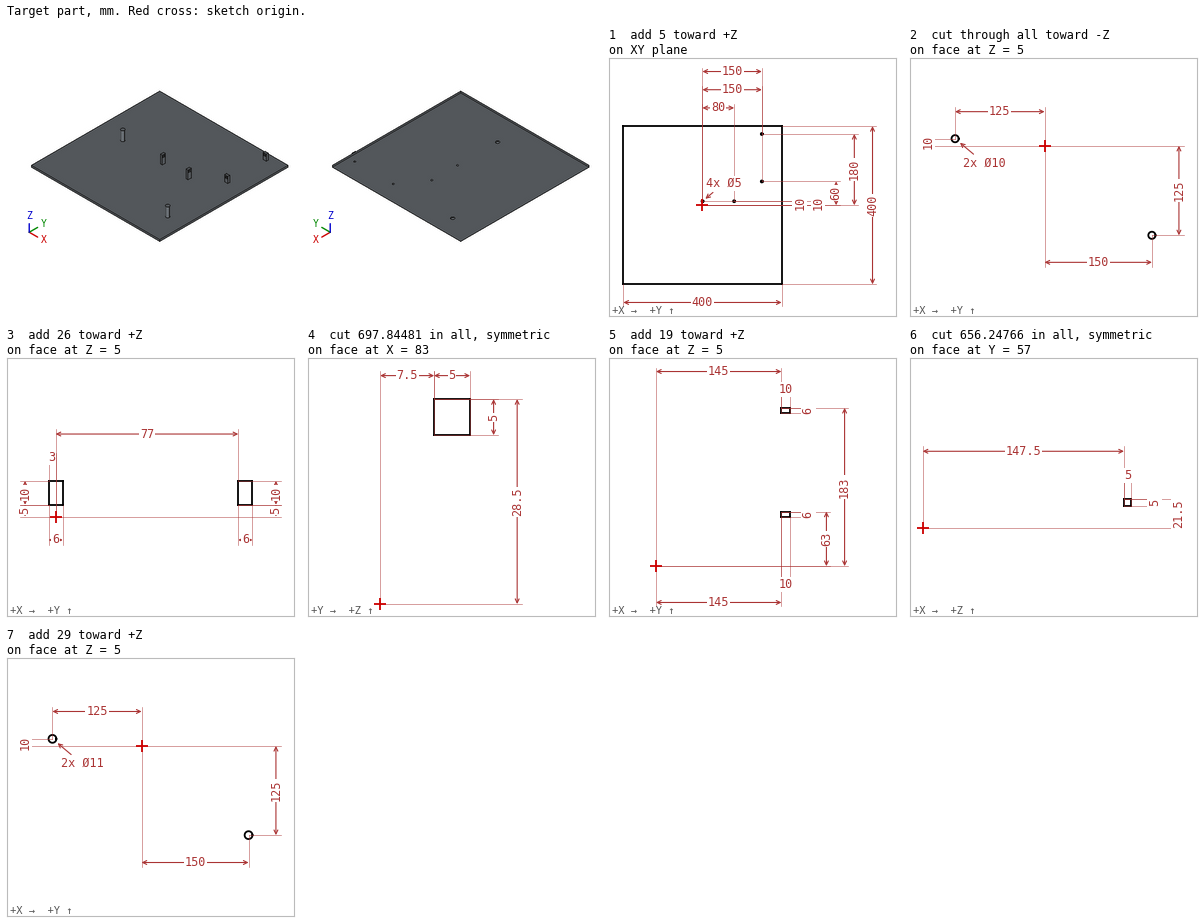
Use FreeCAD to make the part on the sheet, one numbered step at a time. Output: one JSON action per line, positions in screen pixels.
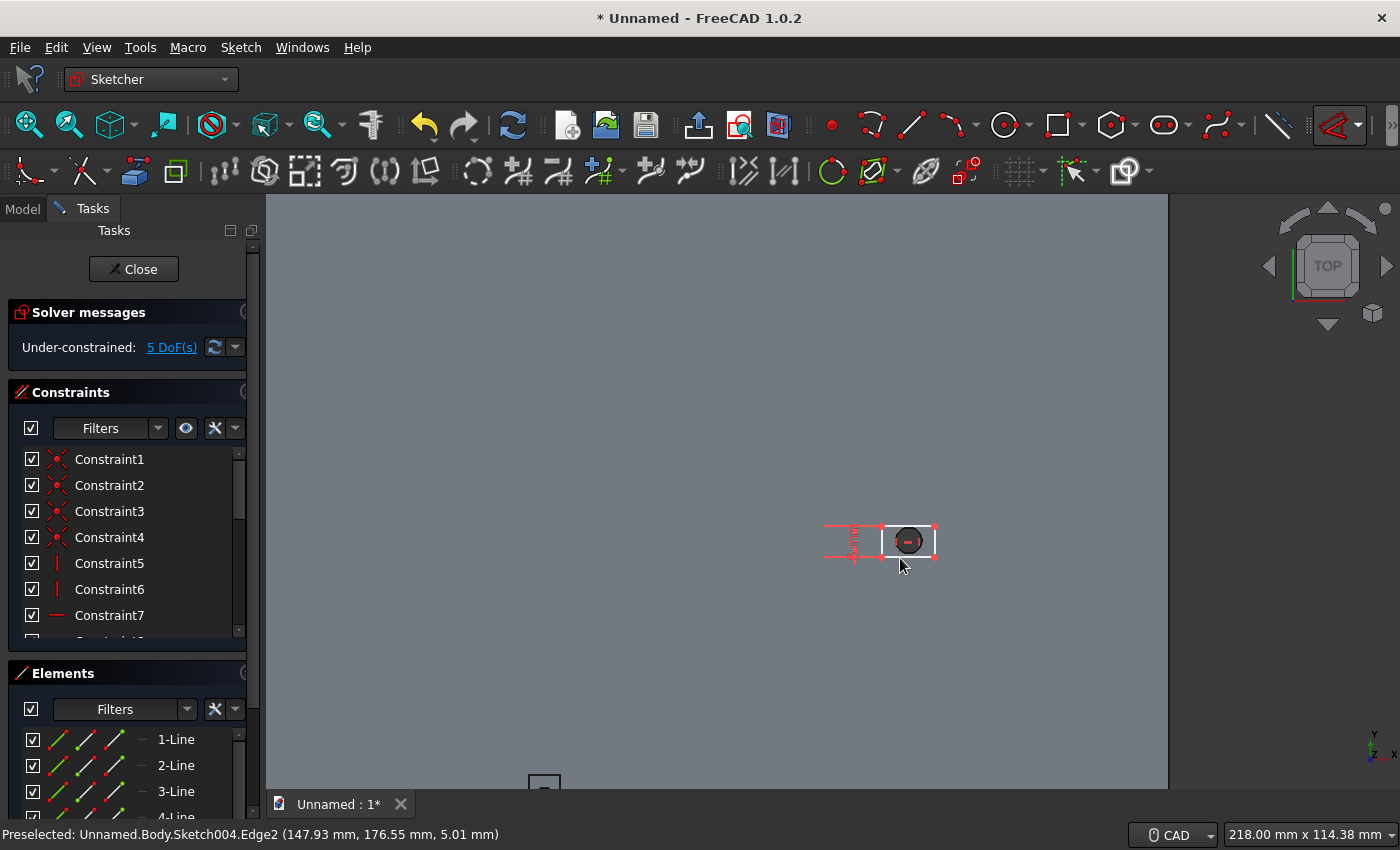
{"action": "left_click", "coordinate": [898, 557]}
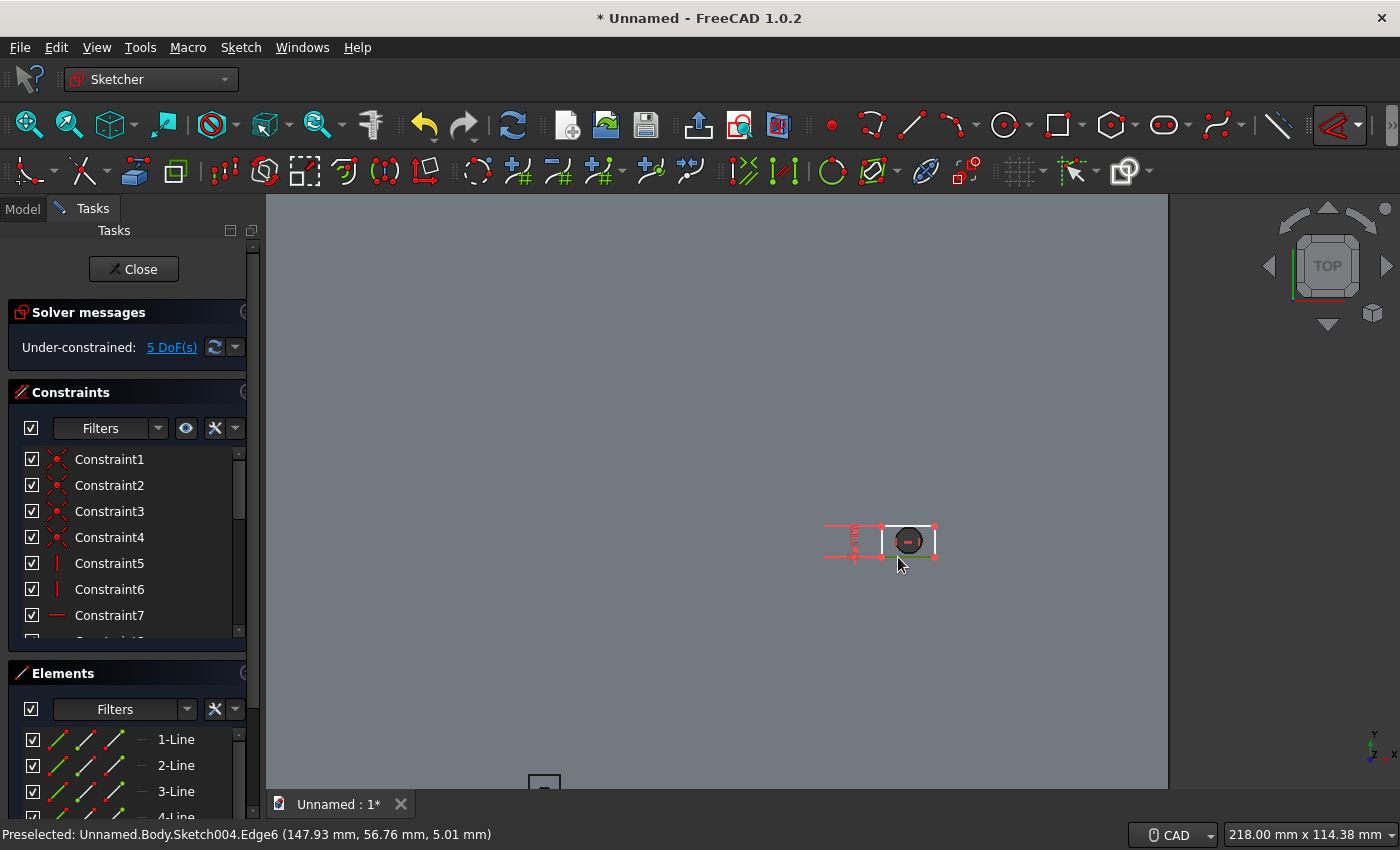
{"action": "key", "text": "l"}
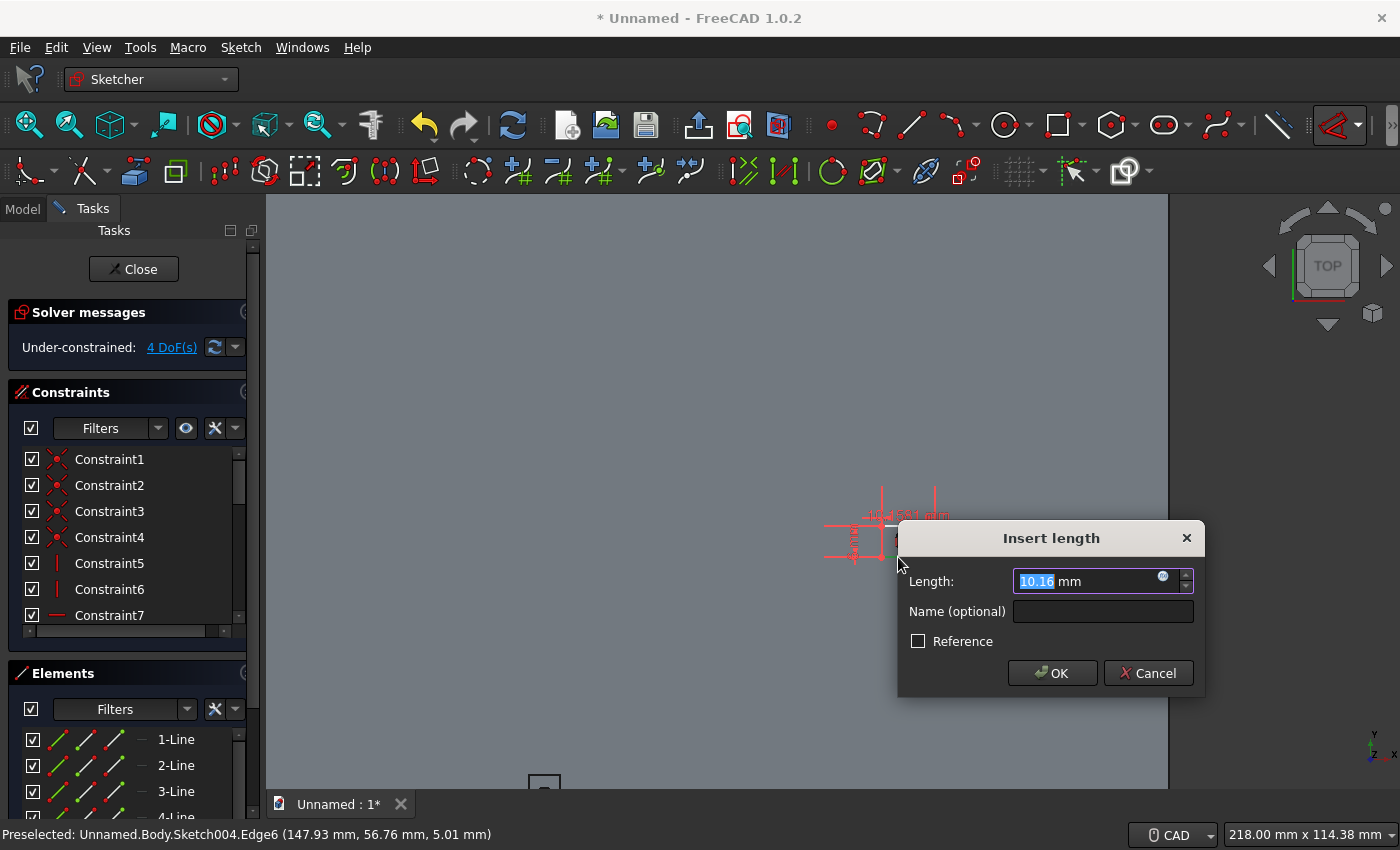
{"action": "type", "text": "10"}
{"action": "key", "text": "Return"}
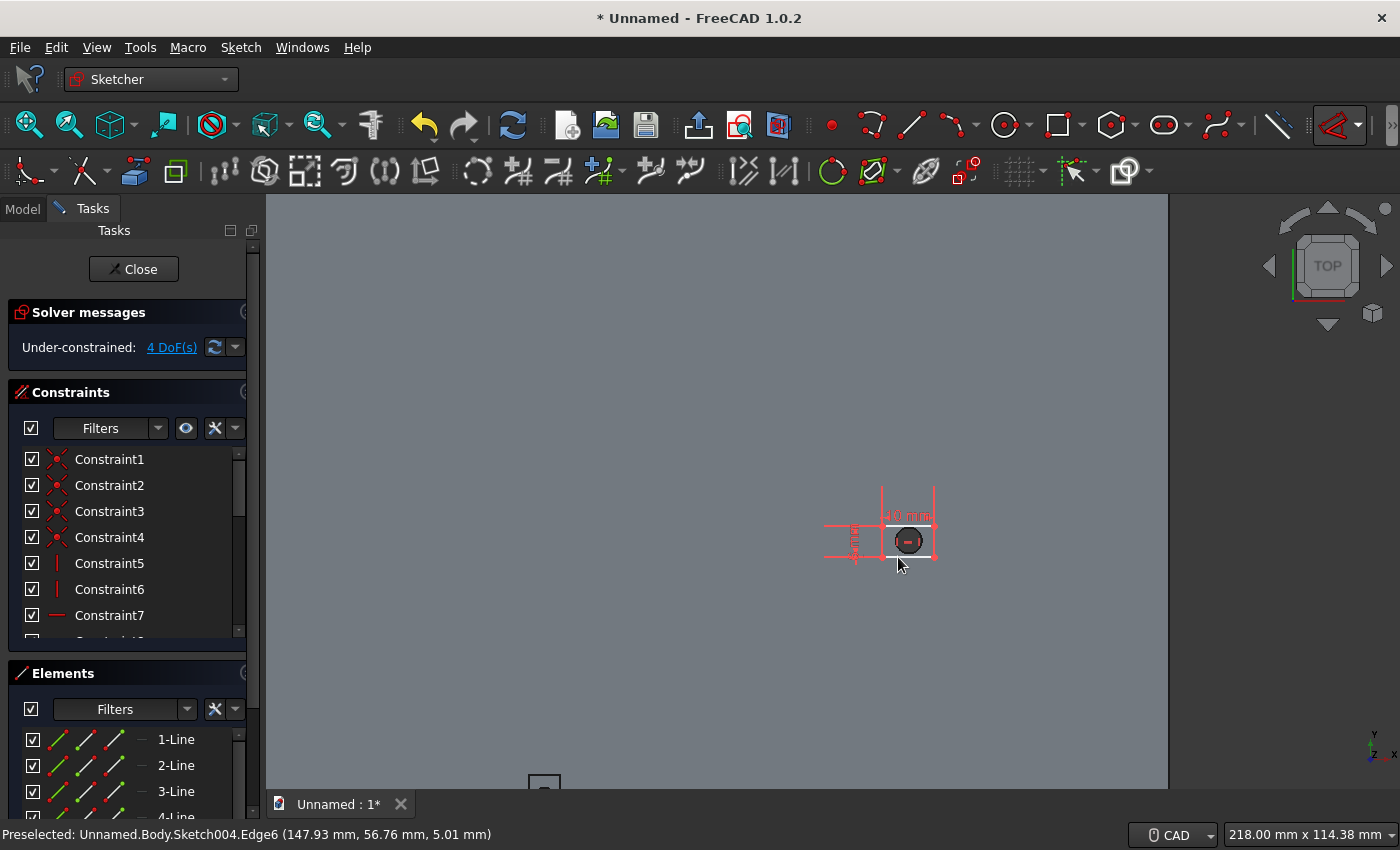
{"action": "left_click", "coordinate": [882, 526]}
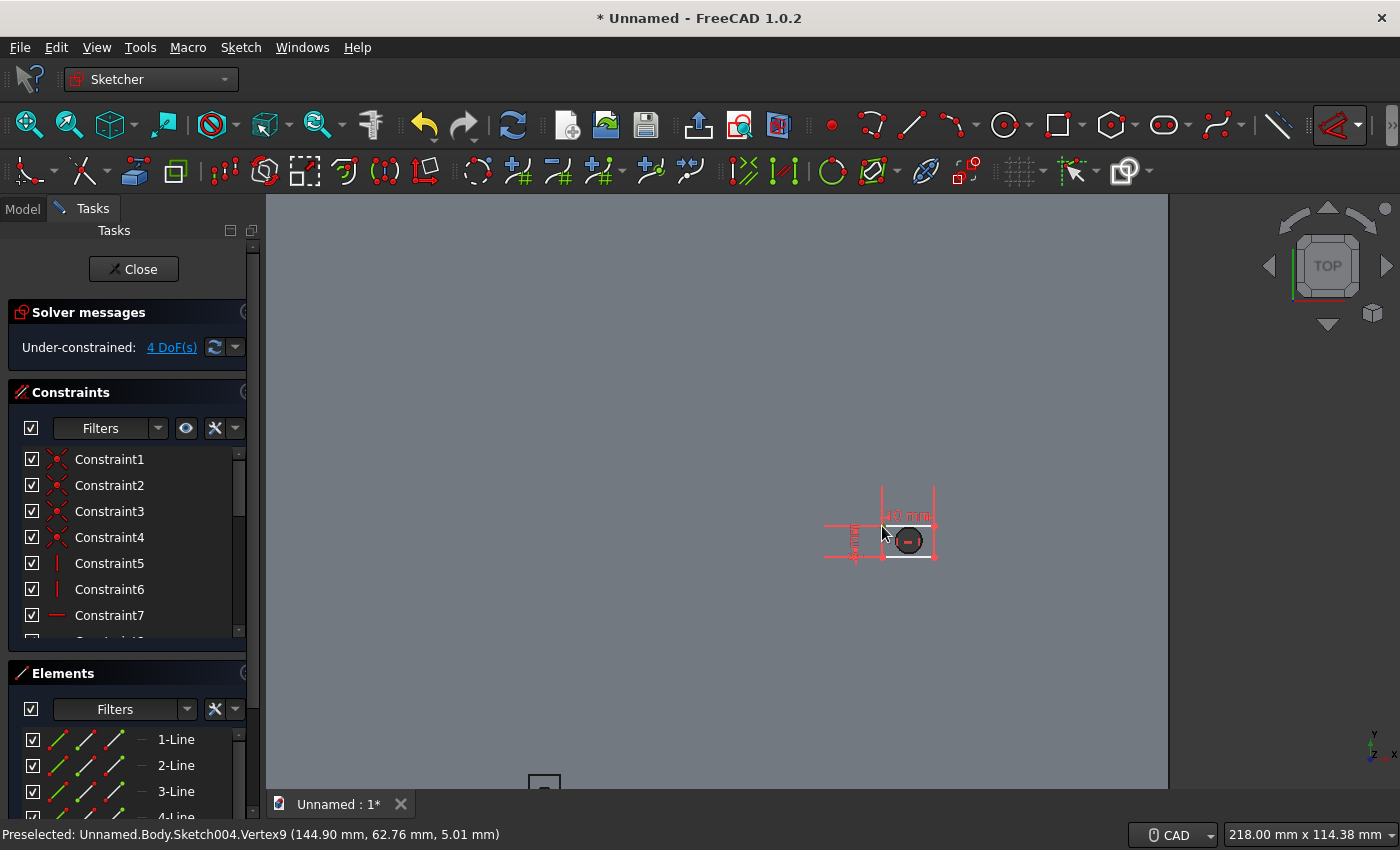
{"action": "key", "text": "i"}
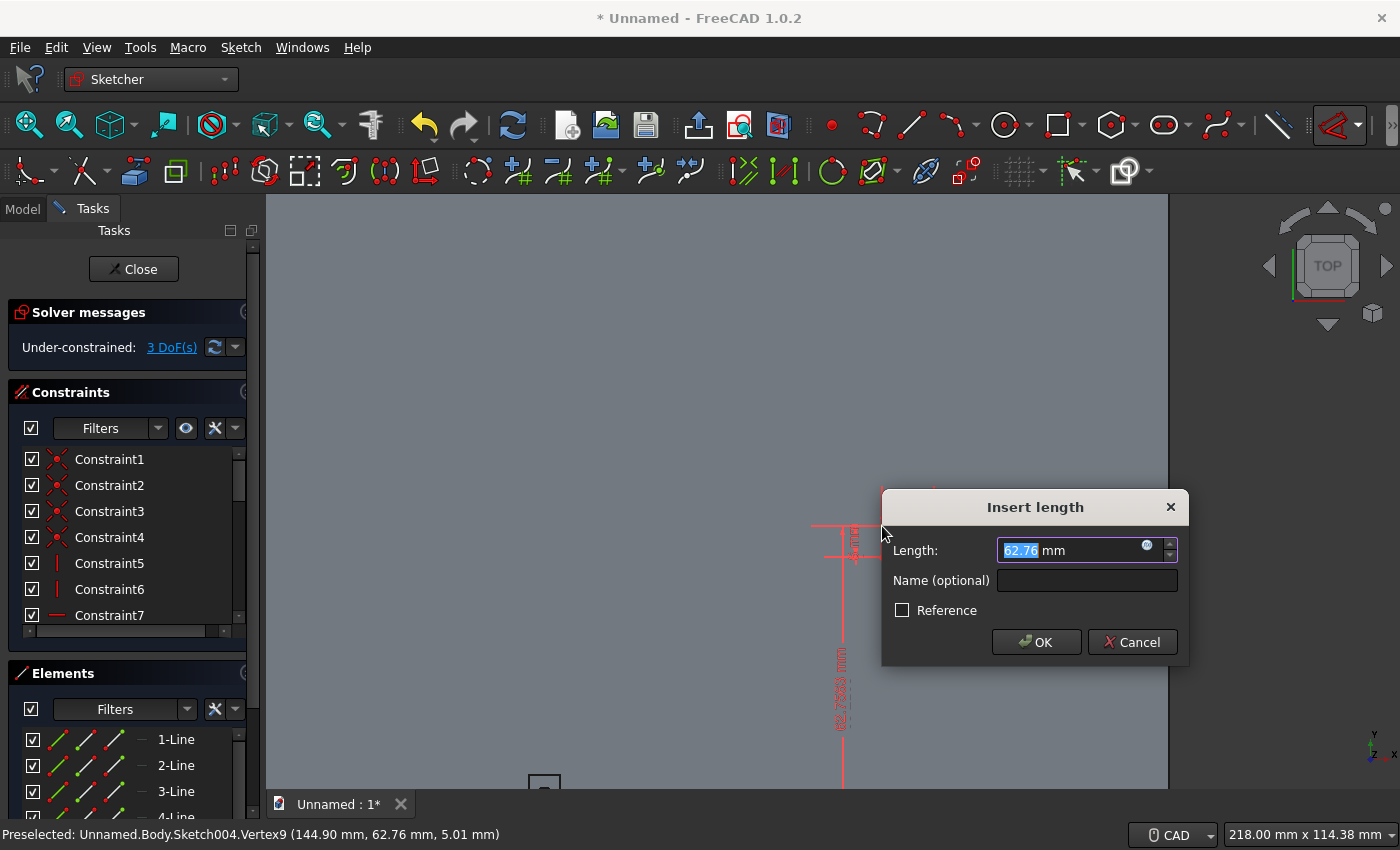
{"action": "type", "text": "63"}
{"action": "key", "text": "Return"}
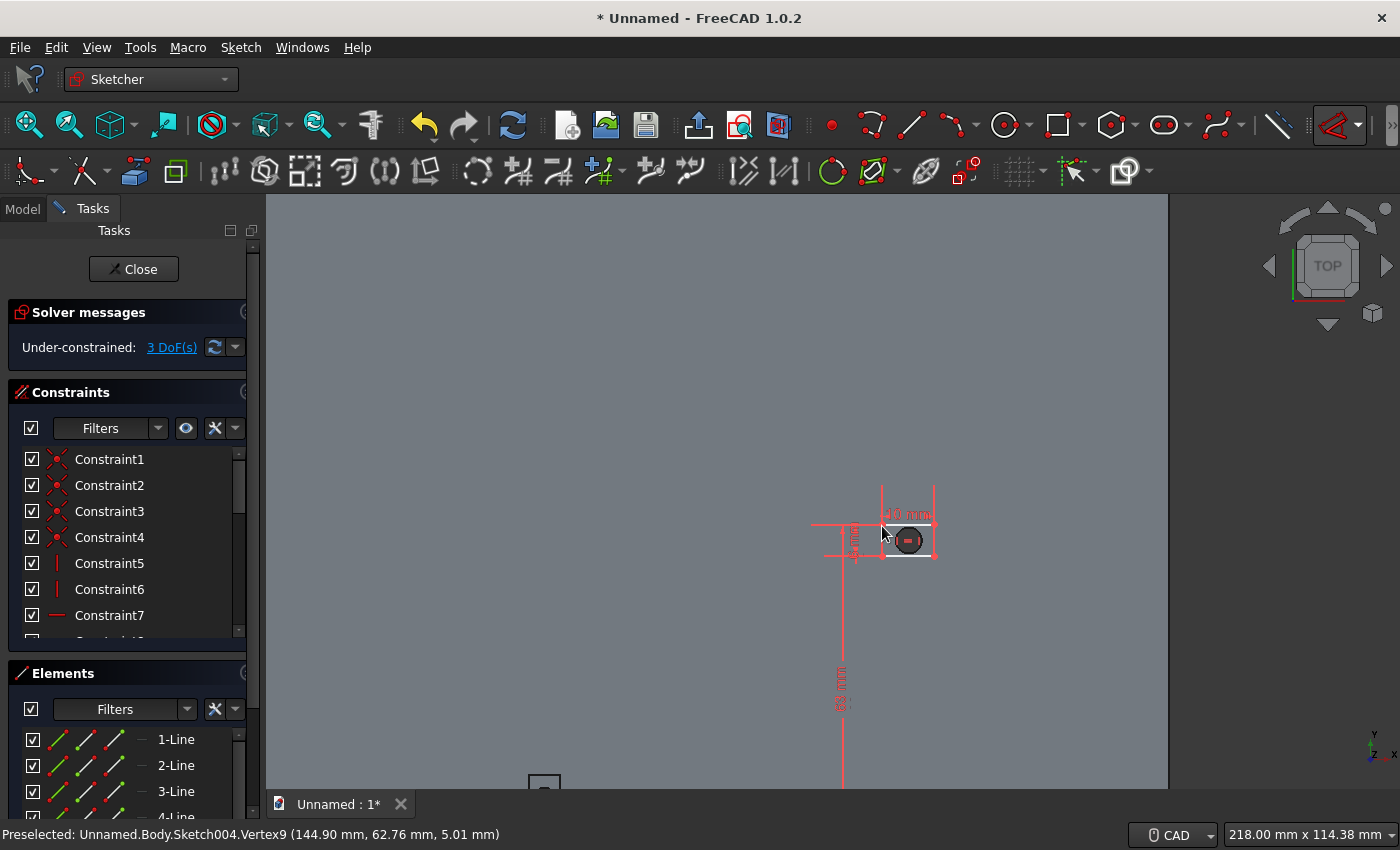
{"action": "scroll", "coordinate": [900, 558], "scroll_direction": "down", "scroll_amount": 5}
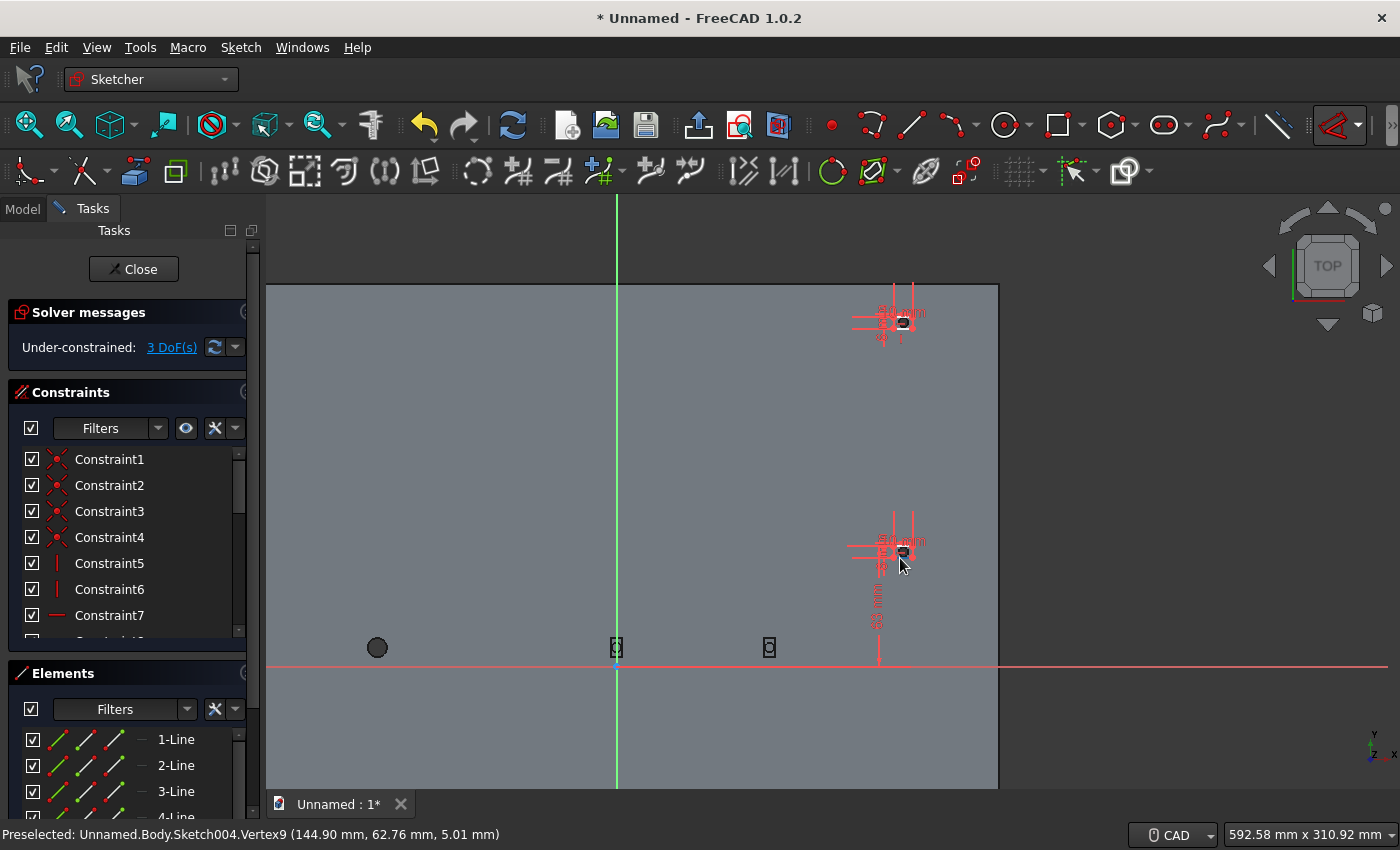
{"action": "left_click", "coordinate": [894, 317]}